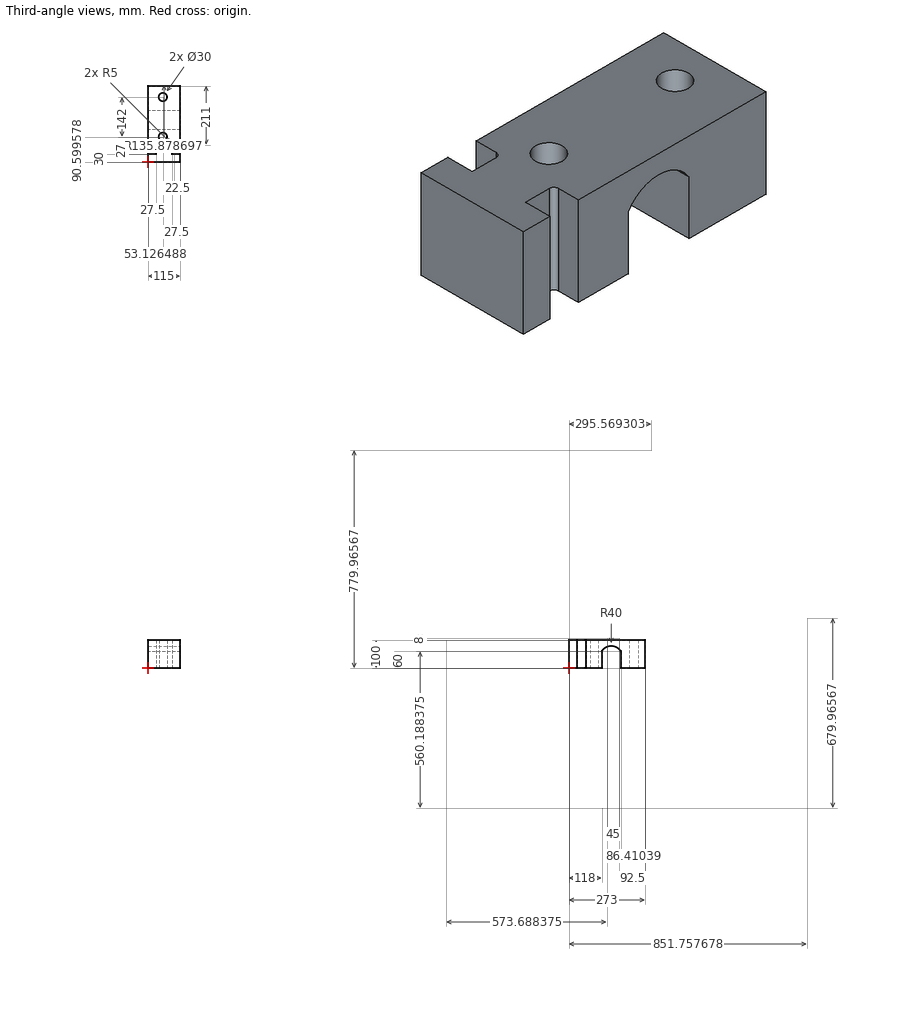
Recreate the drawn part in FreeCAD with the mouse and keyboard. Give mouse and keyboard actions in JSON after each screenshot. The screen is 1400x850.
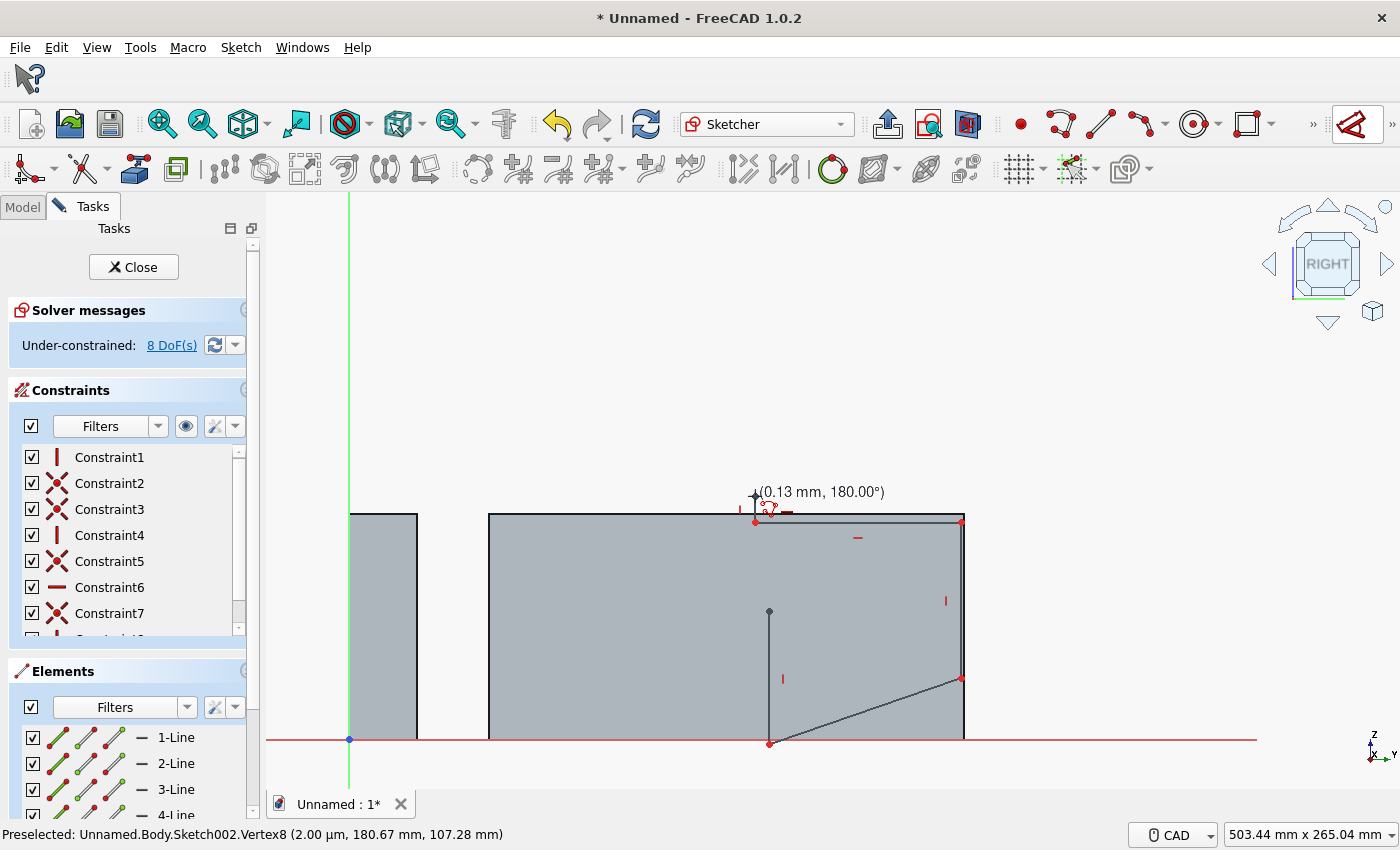
{"action": "scroll", "coordinate": [757, 501], "scroll_direction": "down", "scroll_amount": 10}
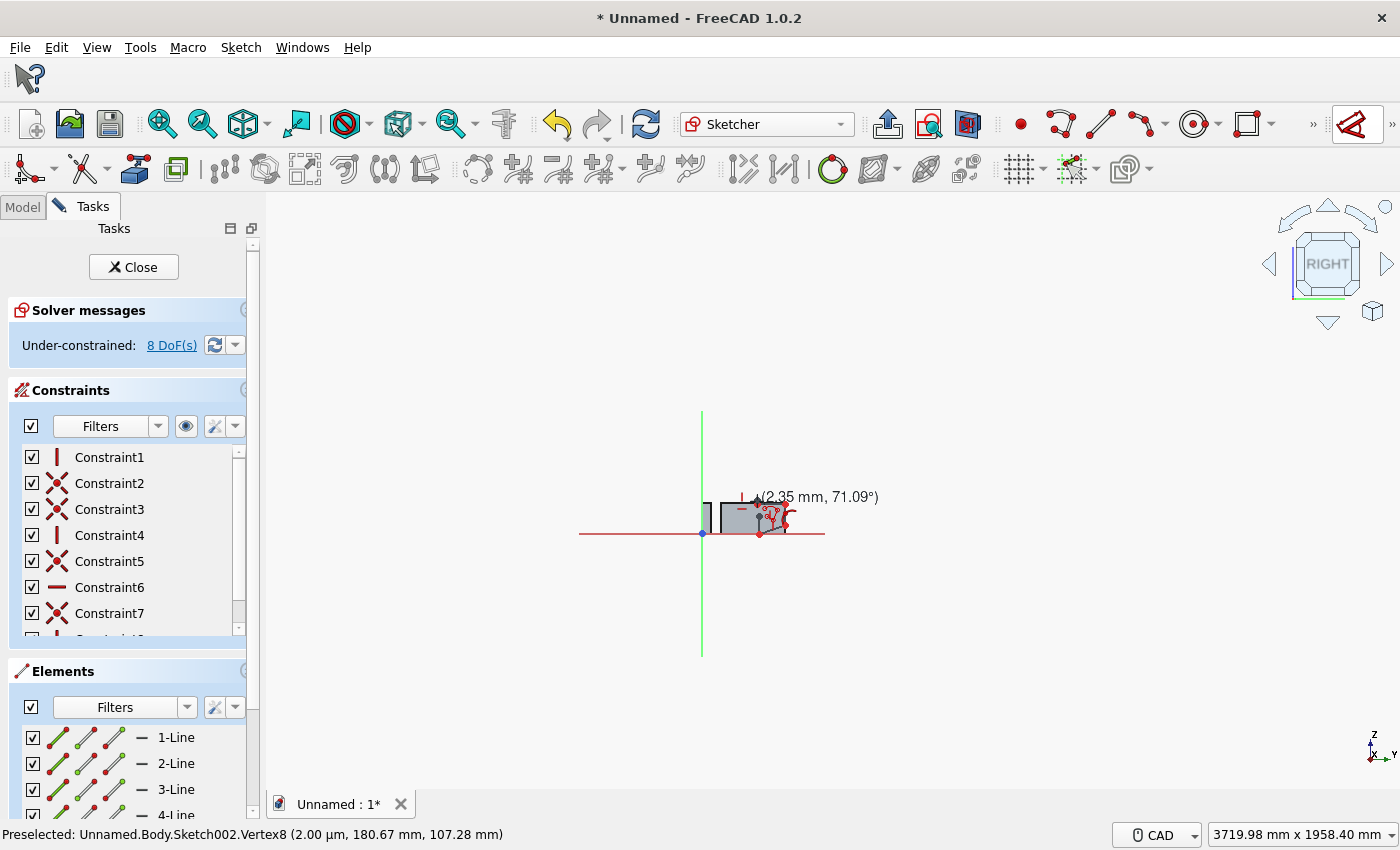
{"action": "left_click", "coordinate": [743, 501]}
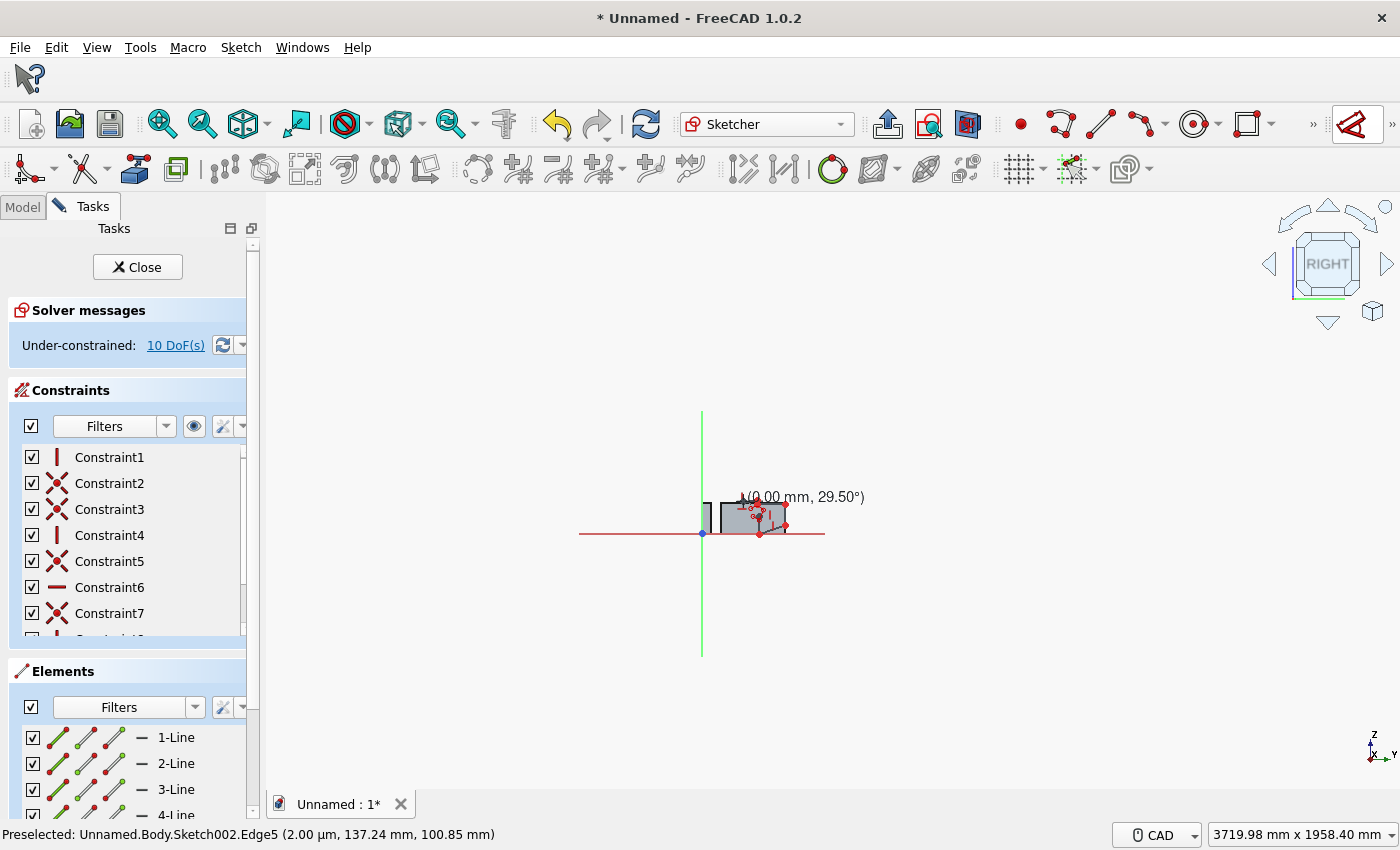
{"action": "scroll", "coordinate": [743, 503], "scroll_direction": "up", "scroll_amount": 10}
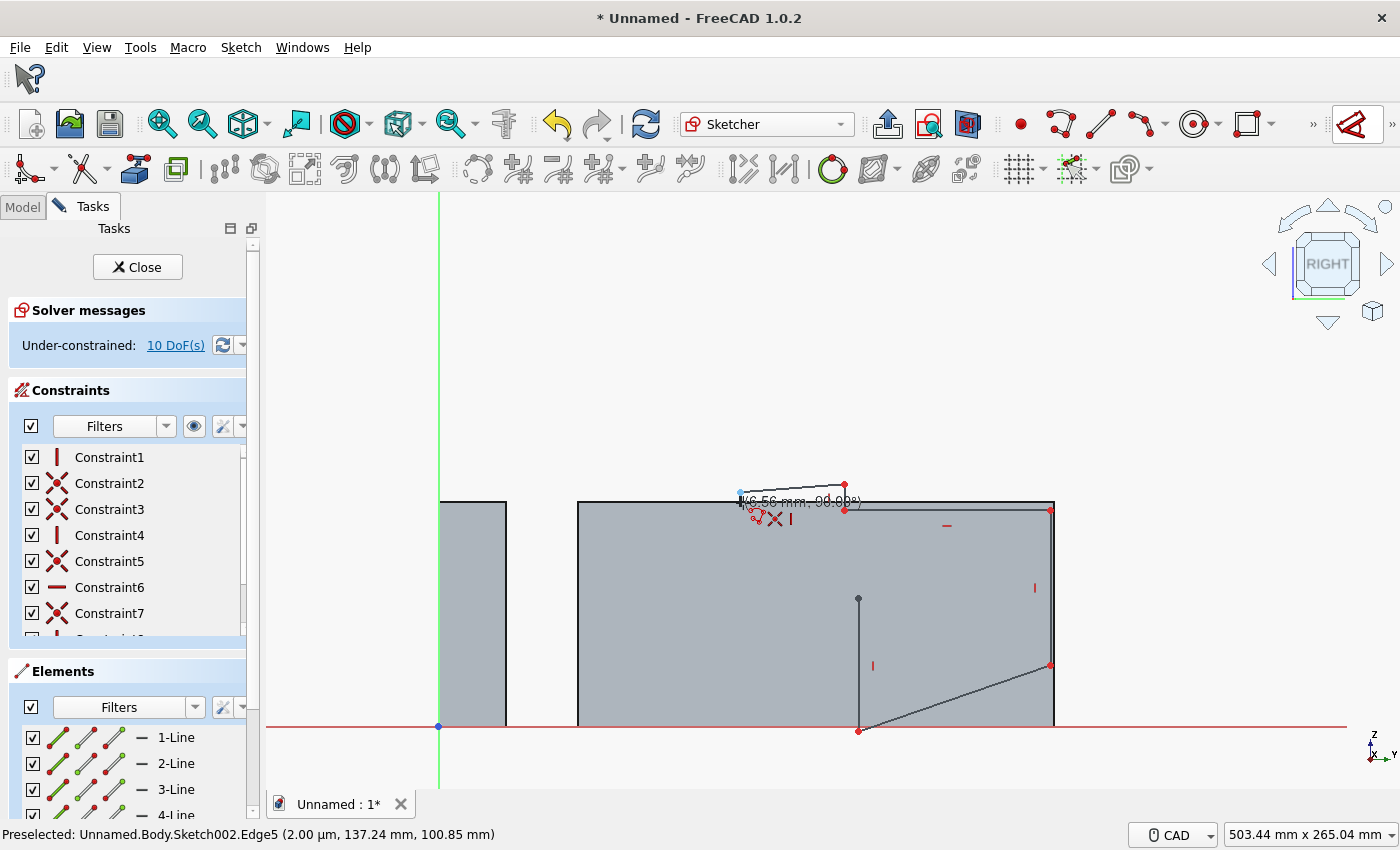
{"action": "left_click", "coordinate": [740, 502]}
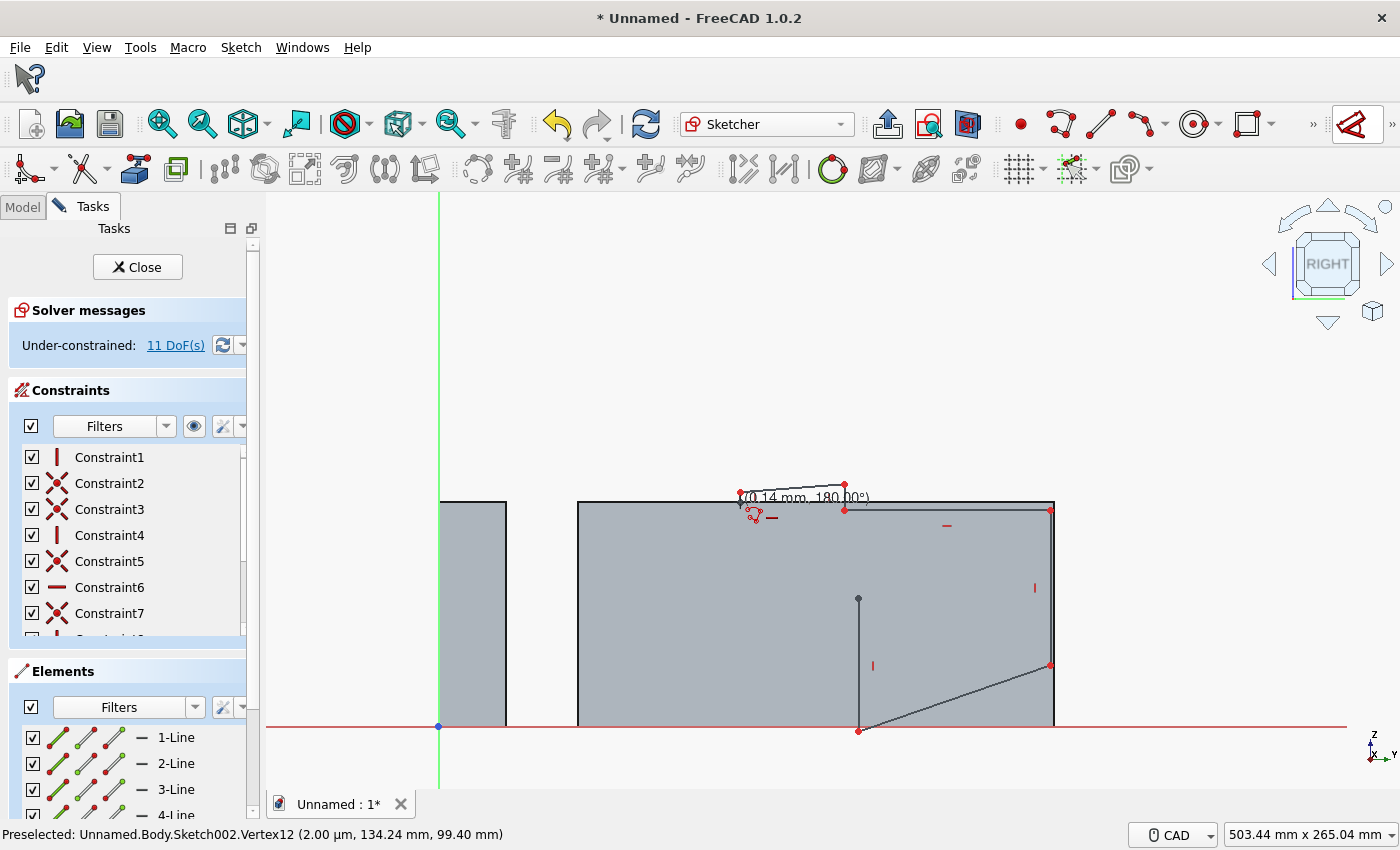
{"action": "scroll", "coordinate": [743, 503], "scroll_direction": "down", "scroll_amount": 10}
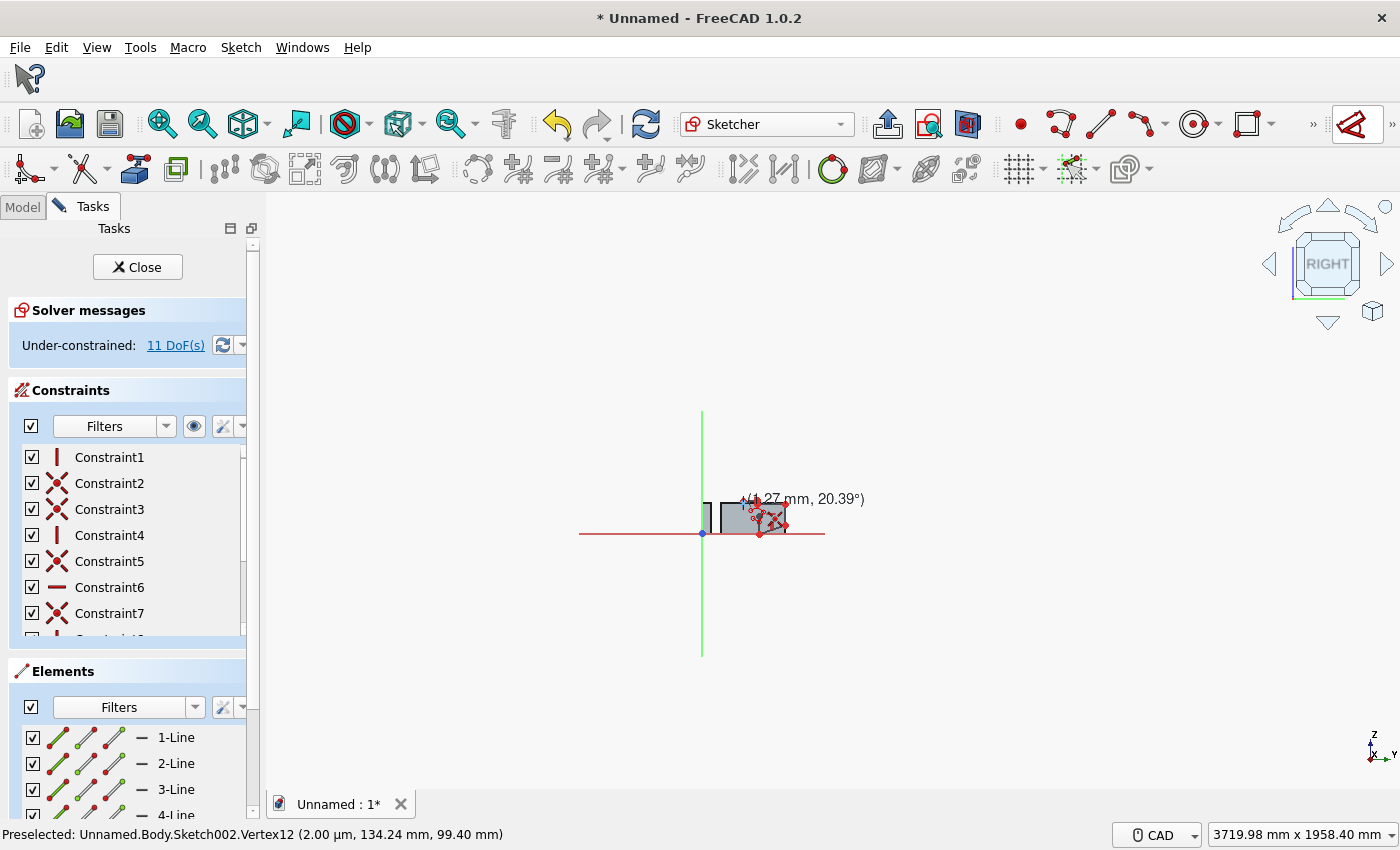
{"action": "left_click", "coordinate": [569, 503]}
{"action": "left_click", "coordinate": [792, 296]}
{"action": "left_click", "coordinate": [962, 479]}
{"action": "left_click", "coordinate": [738, 686]}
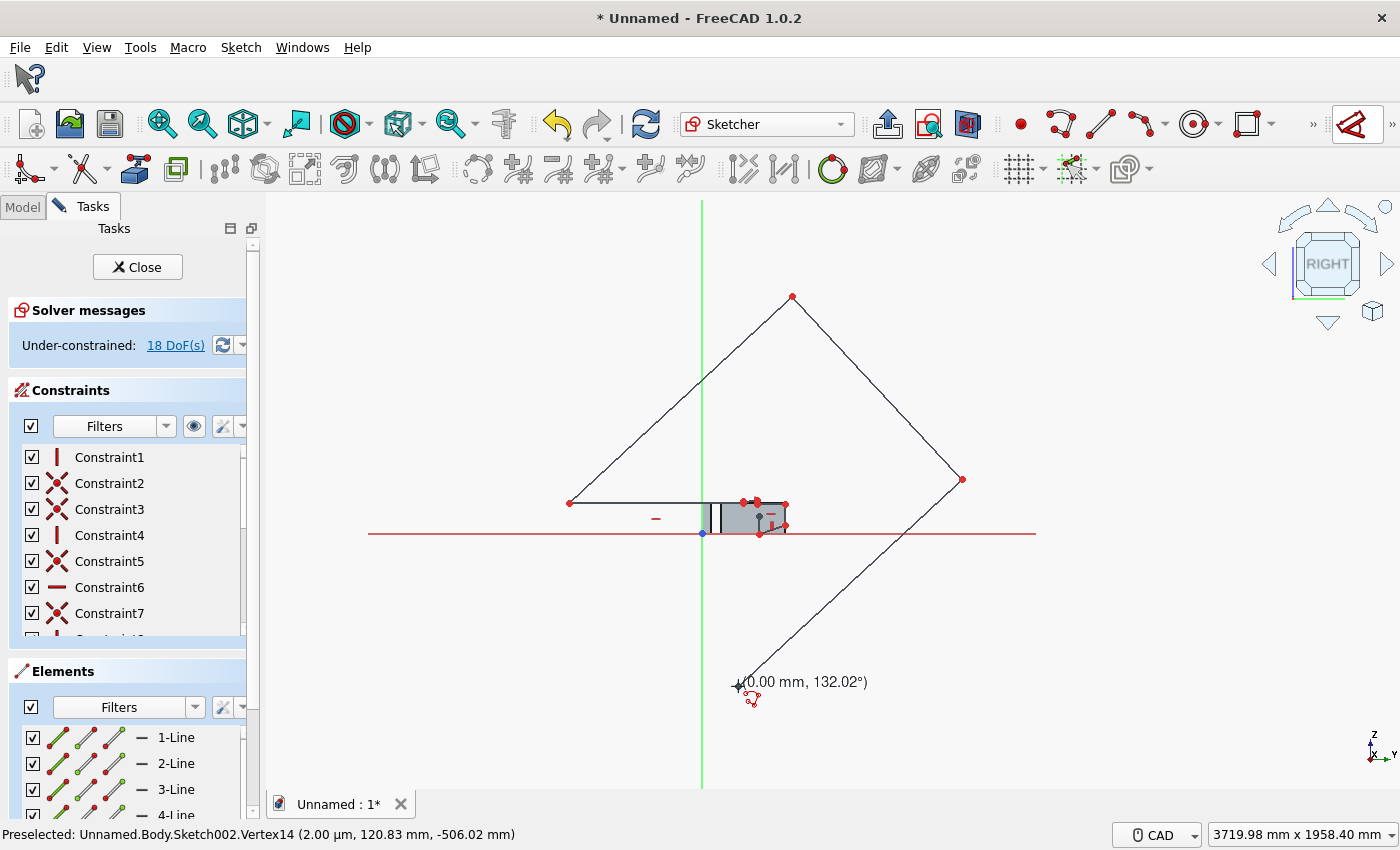
{"action": "scroll", "coordinate": [738, 515], "scroll_direction": "up", "scroll_amount": 2}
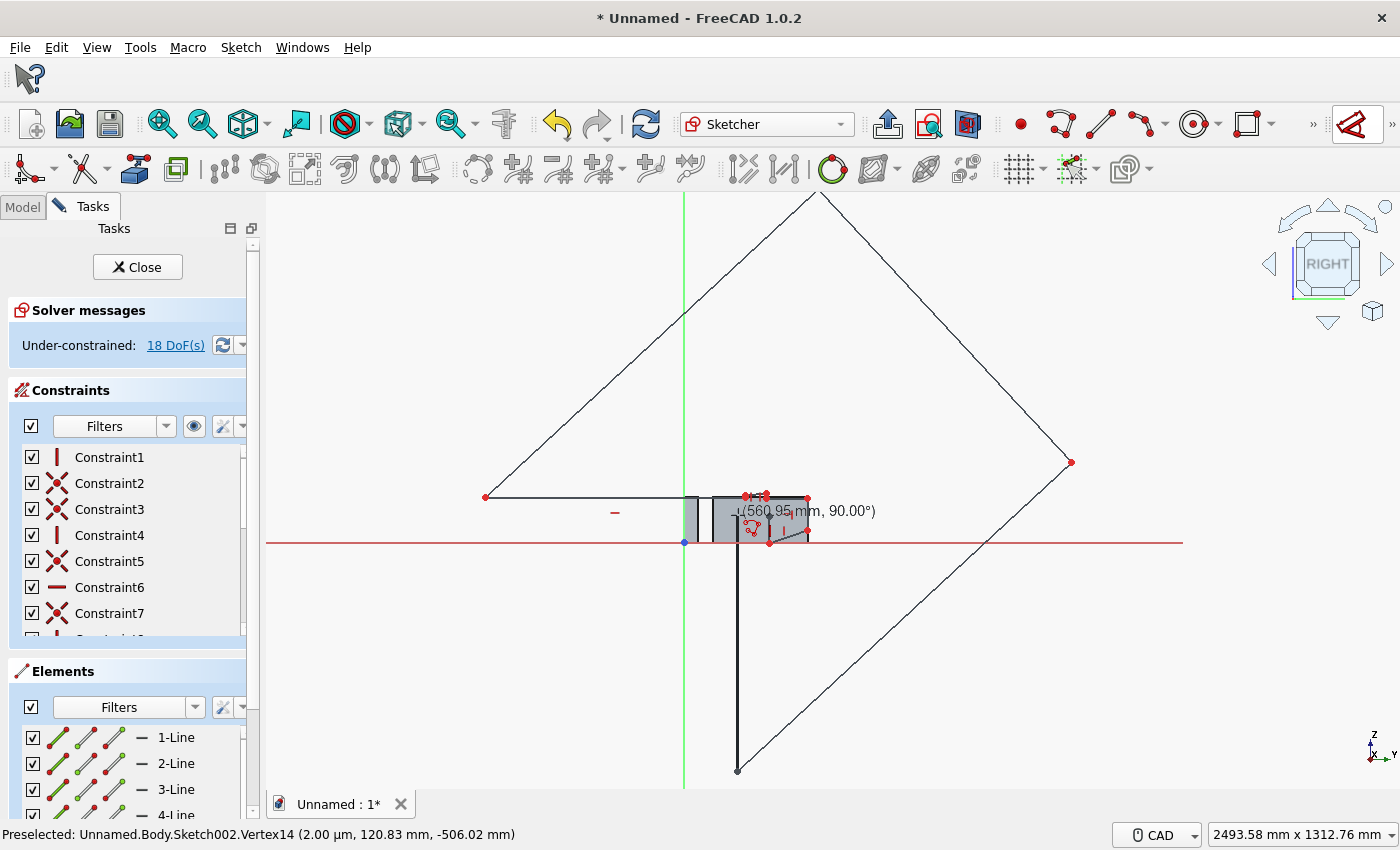
{"action": "left_click", "coordinate": [738, 515]}
{"action": "right_click", "coordinate": [738, 515]}